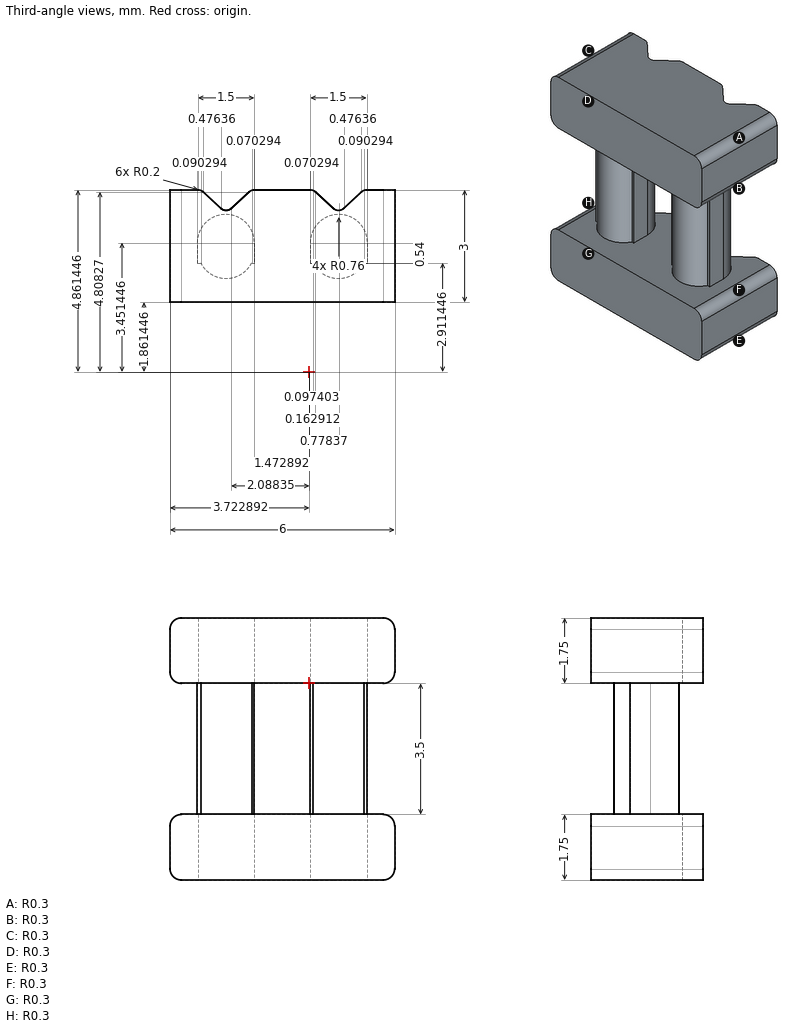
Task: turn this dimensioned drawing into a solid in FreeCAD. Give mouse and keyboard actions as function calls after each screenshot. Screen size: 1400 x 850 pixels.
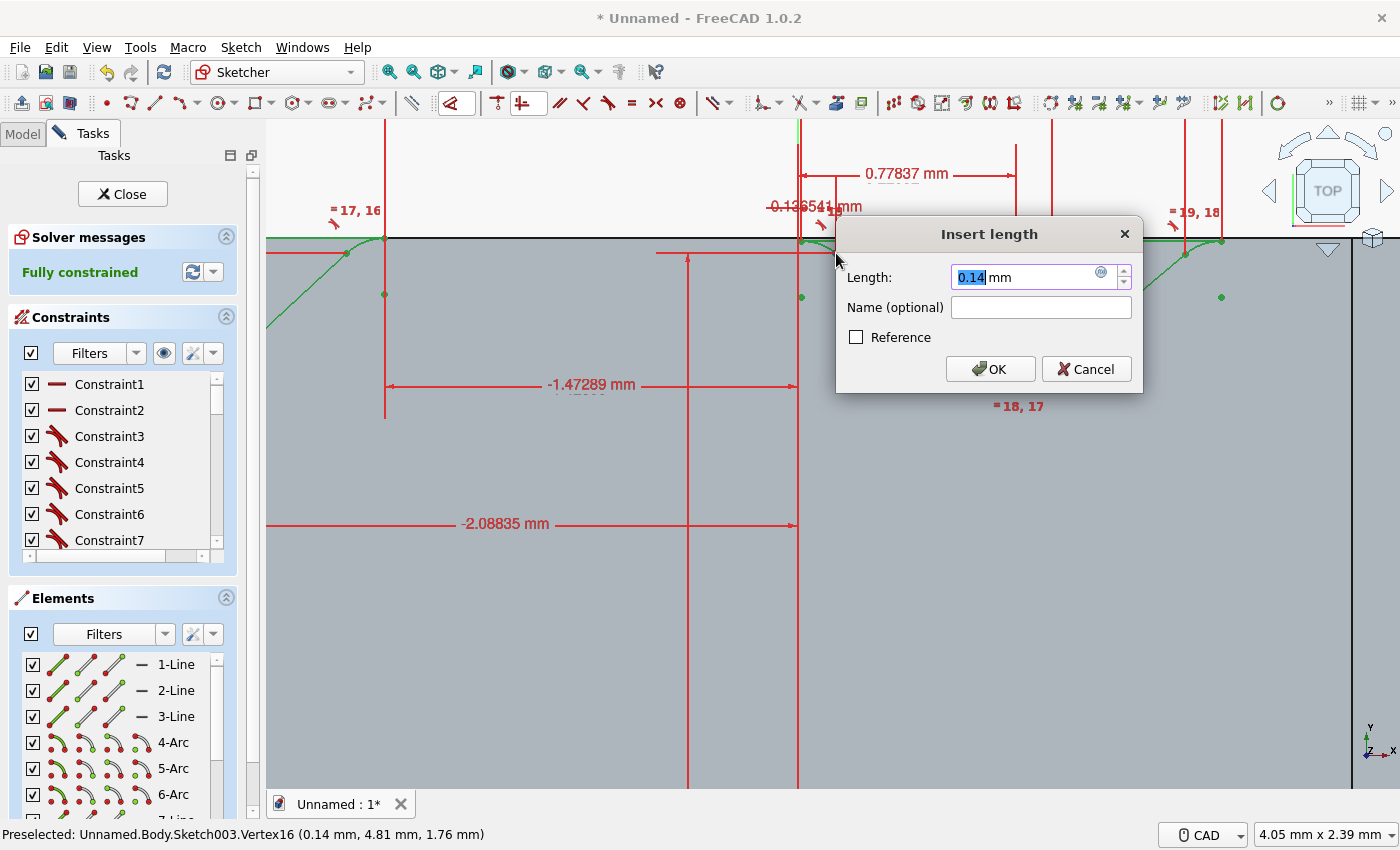
text(0.162912)
key(Return)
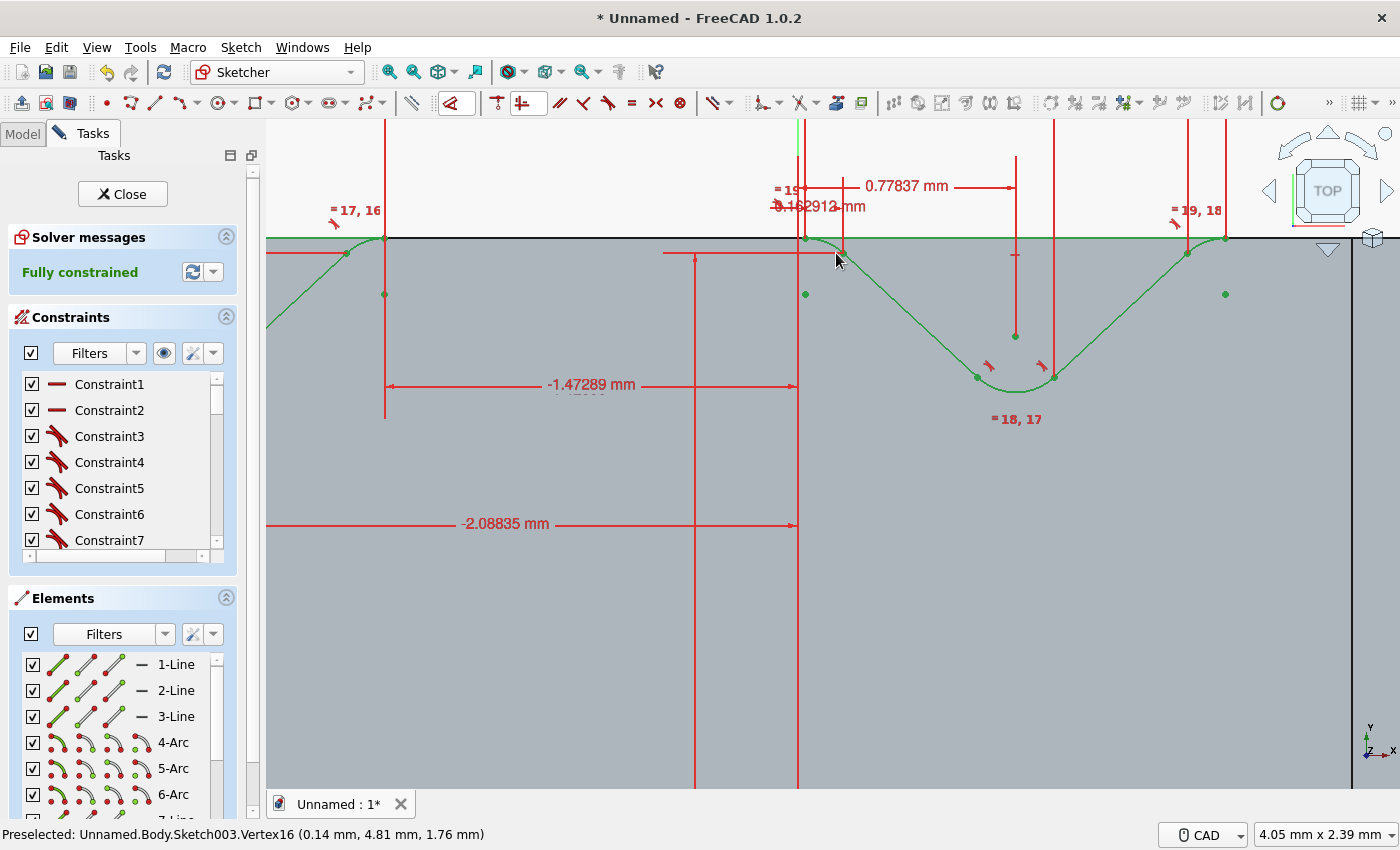
click(123, 194)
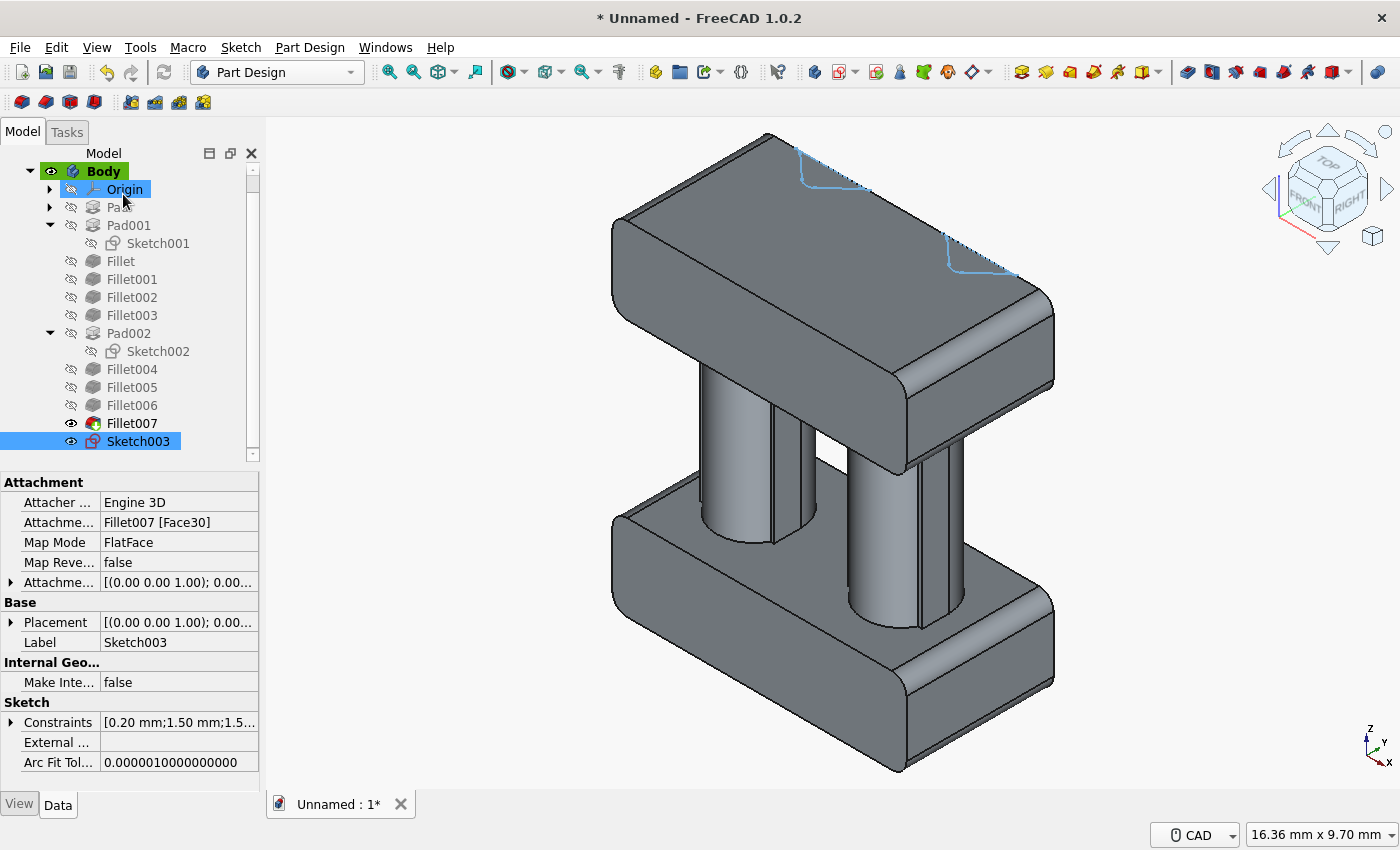
click(1188, 72)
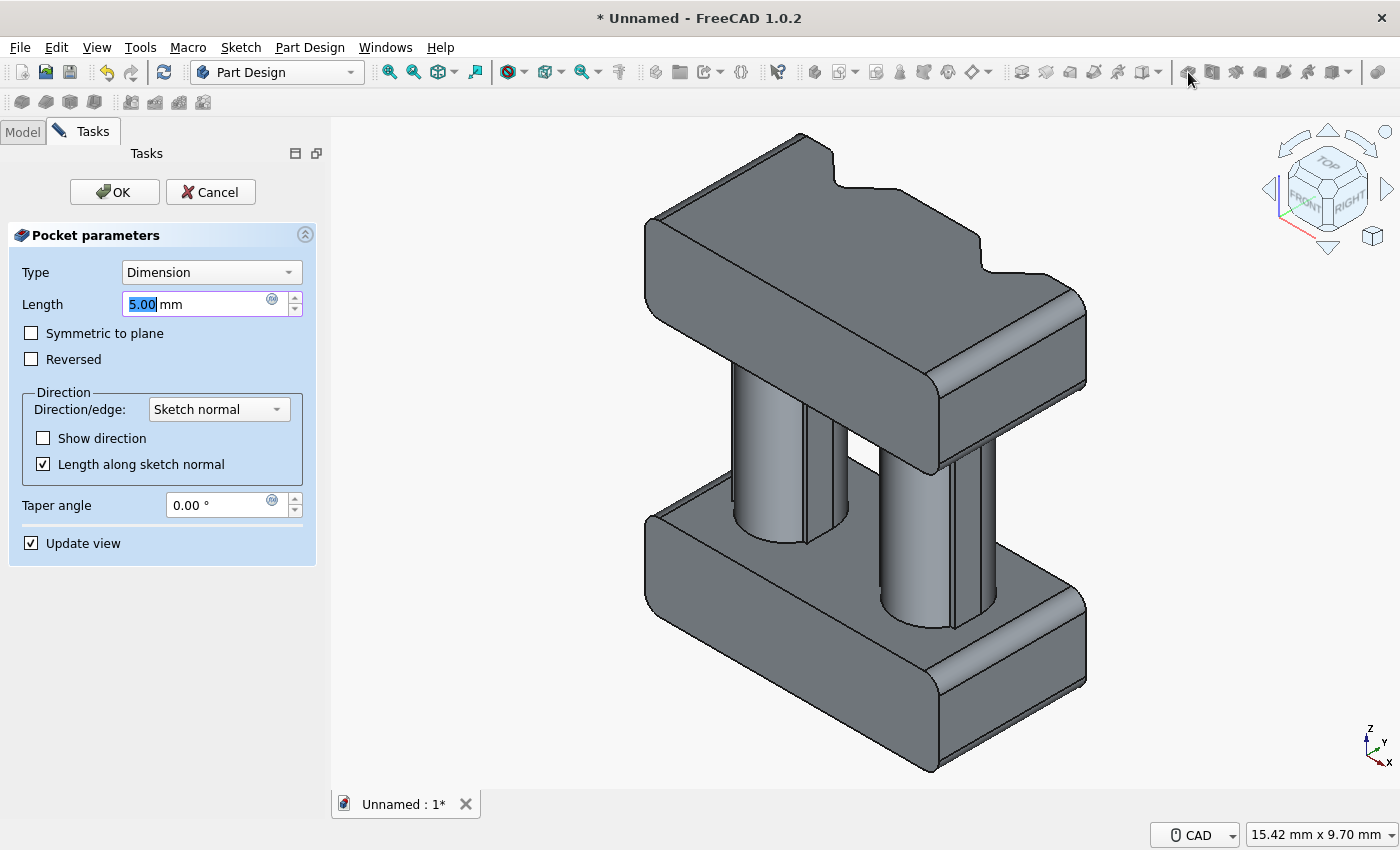
click(212, 272)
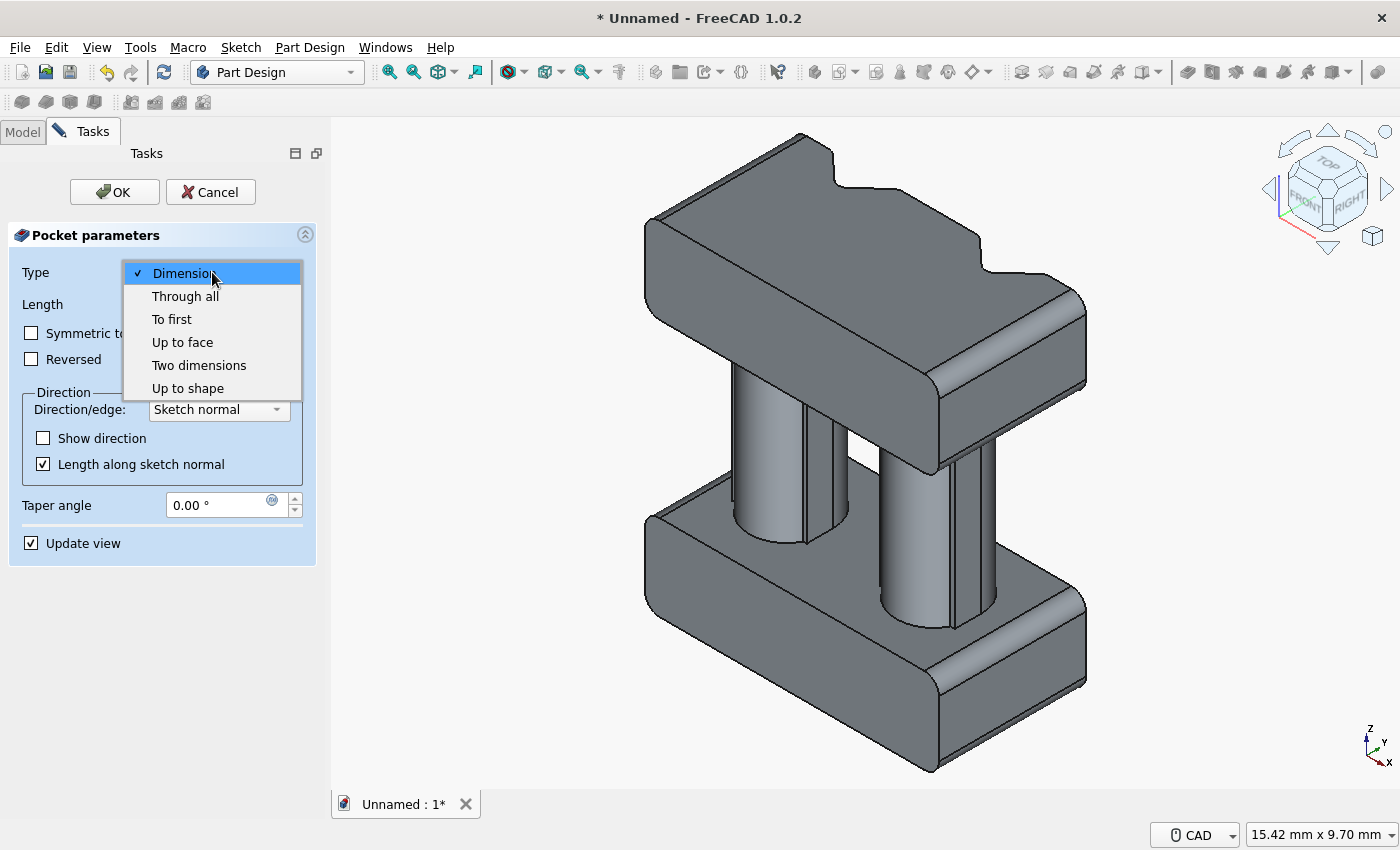
click(212, 296)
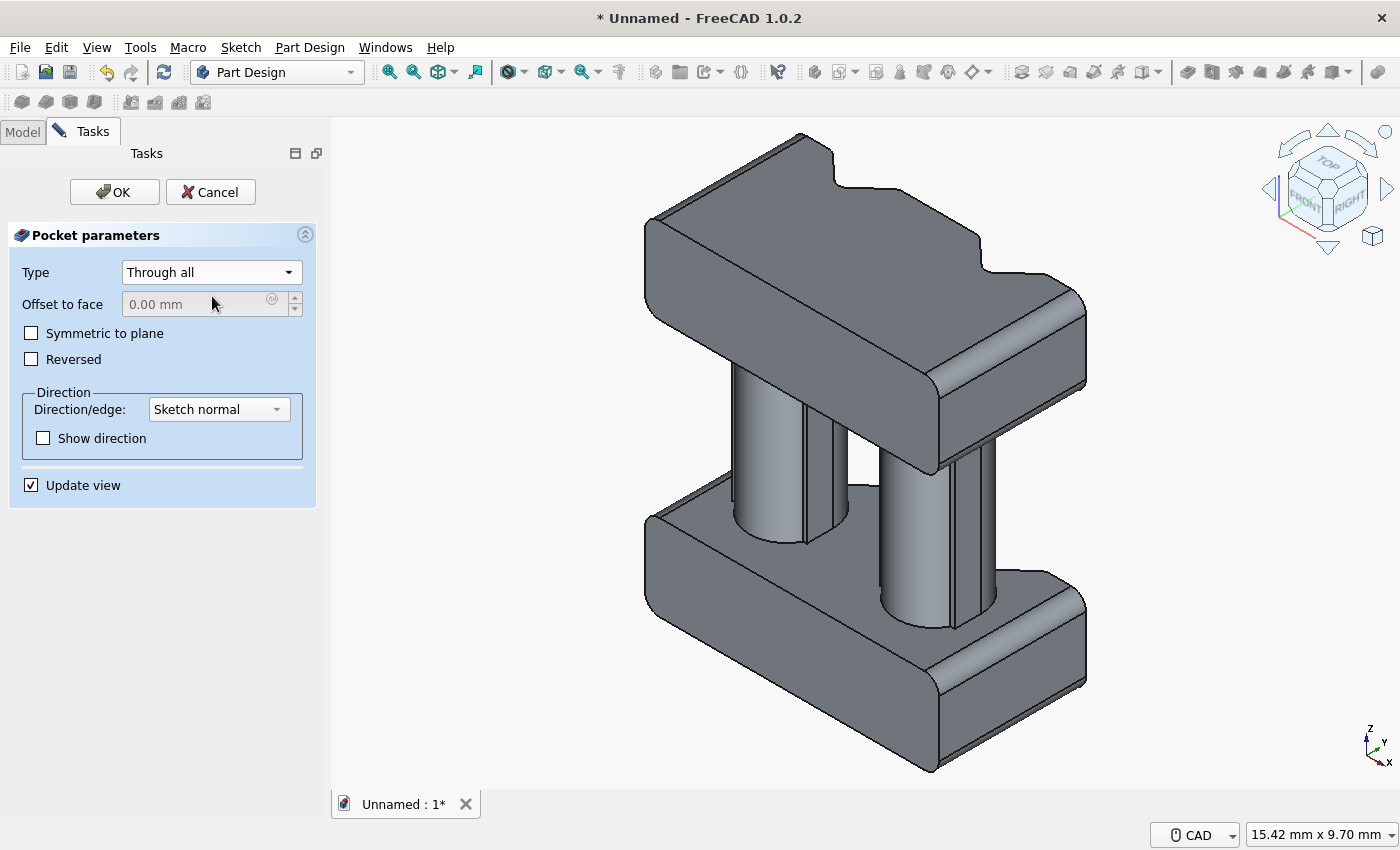
click(115, 192)